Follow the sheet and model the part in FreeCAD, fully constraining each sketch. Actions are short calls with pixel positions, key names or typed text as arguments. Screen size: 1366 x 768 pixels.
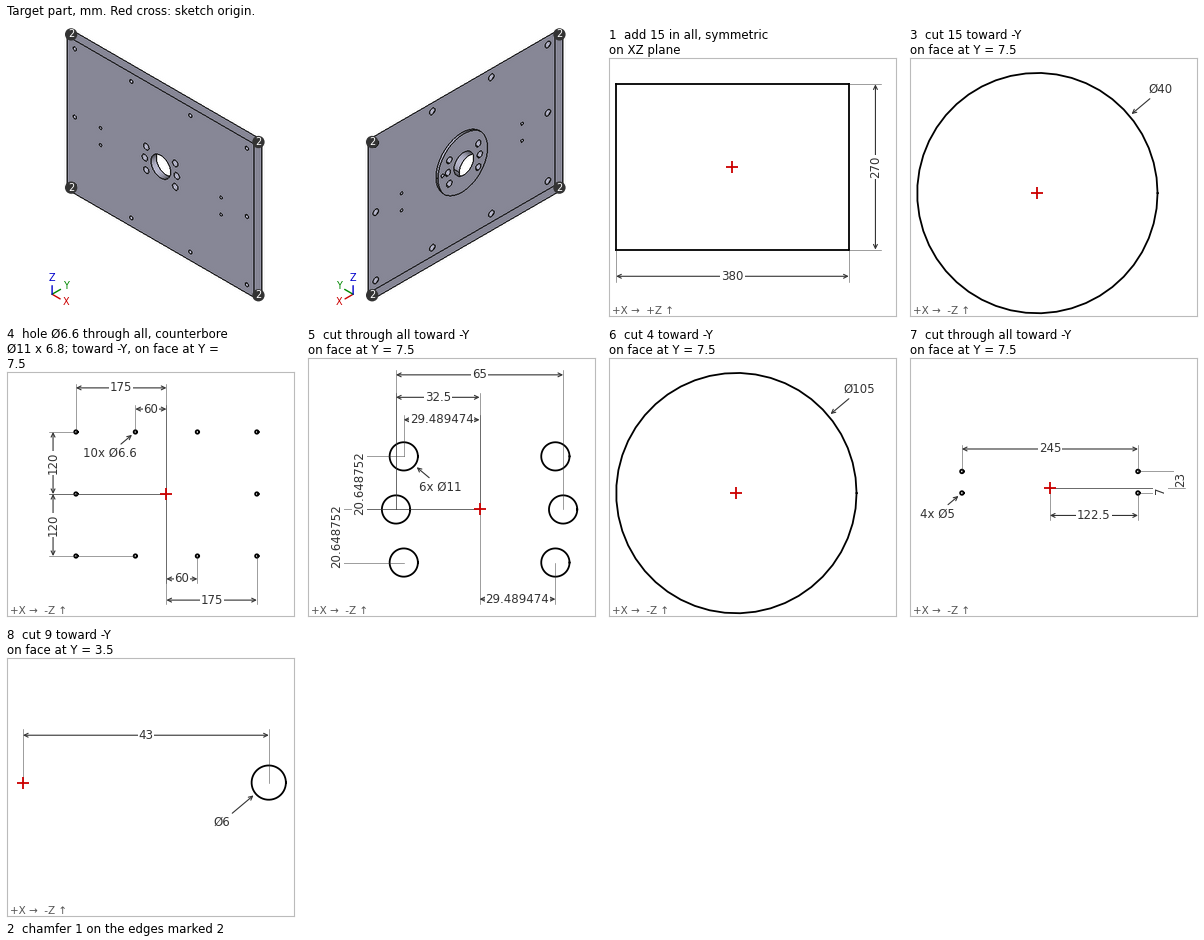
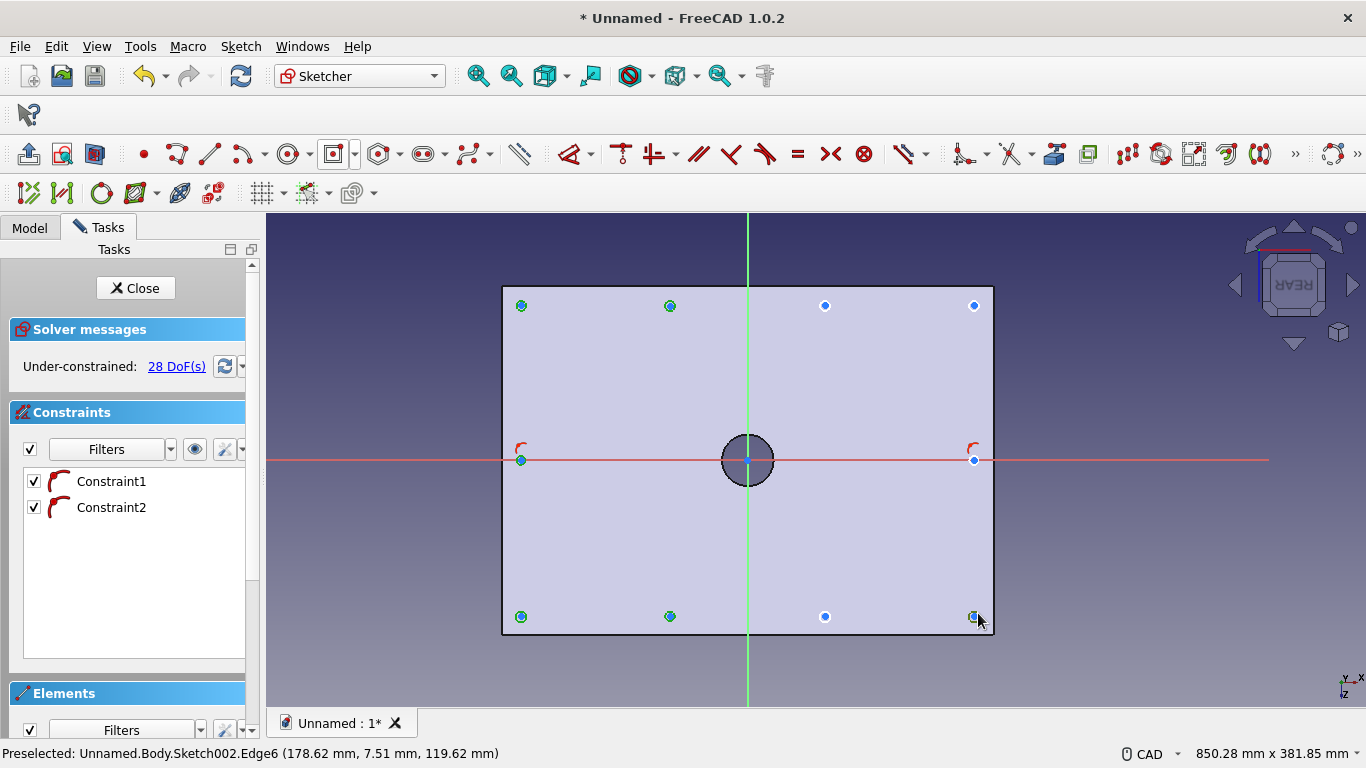
scroll(974, 456, up, 6)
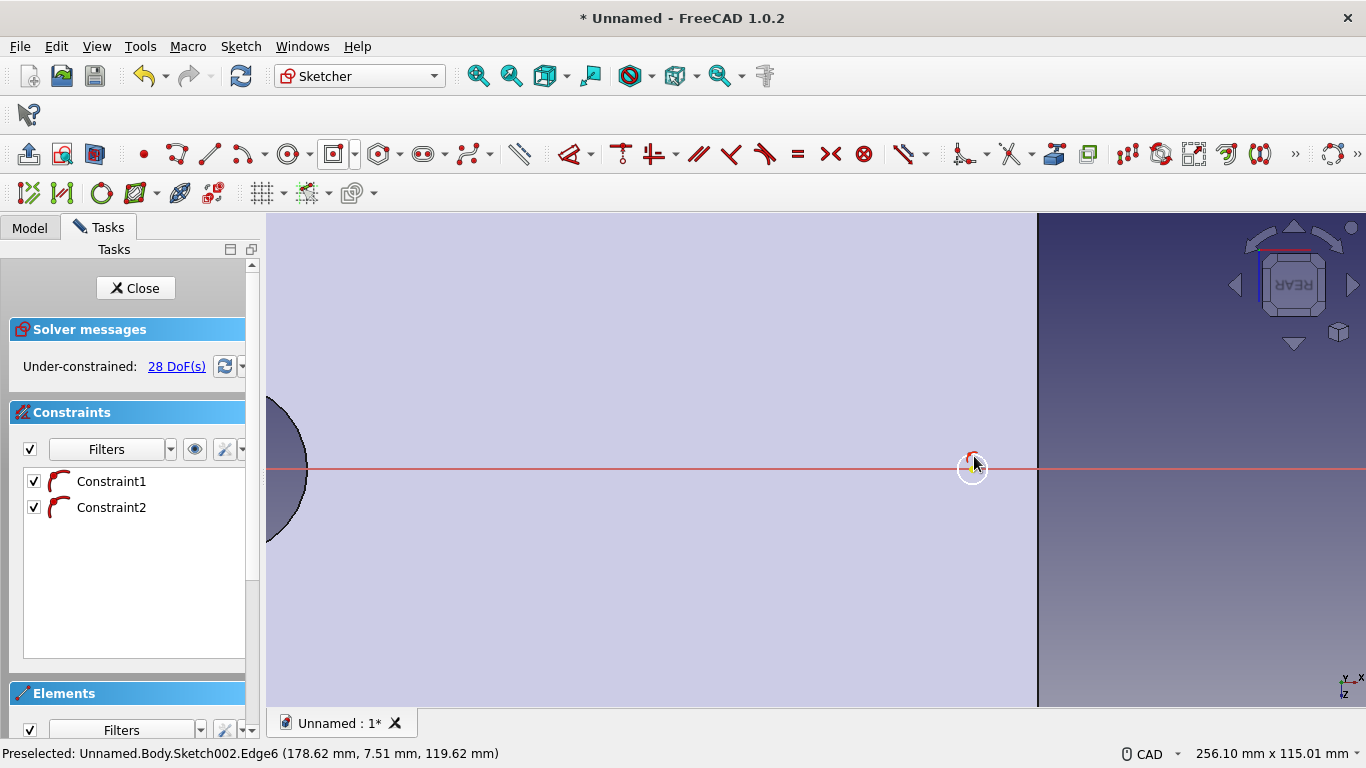
click(958, 469)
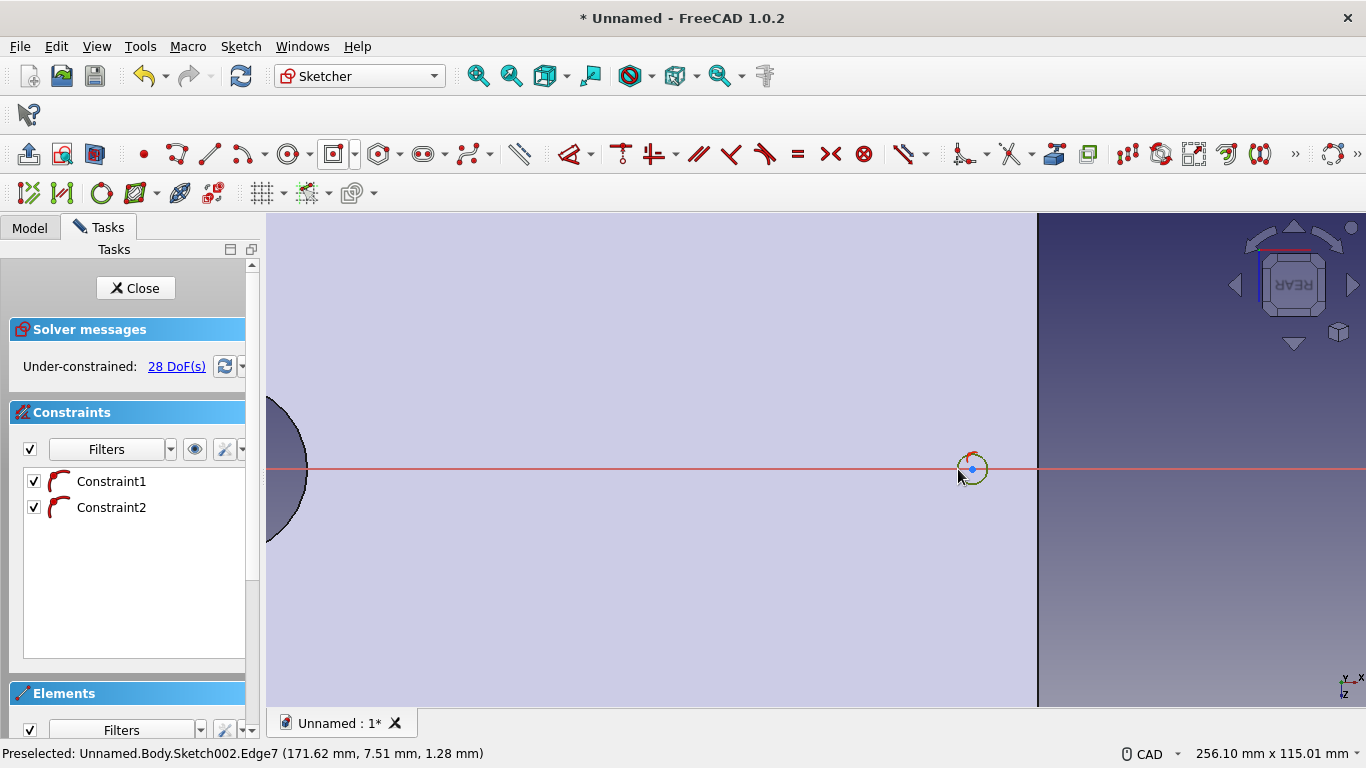
scroll(974, 456, down, 6)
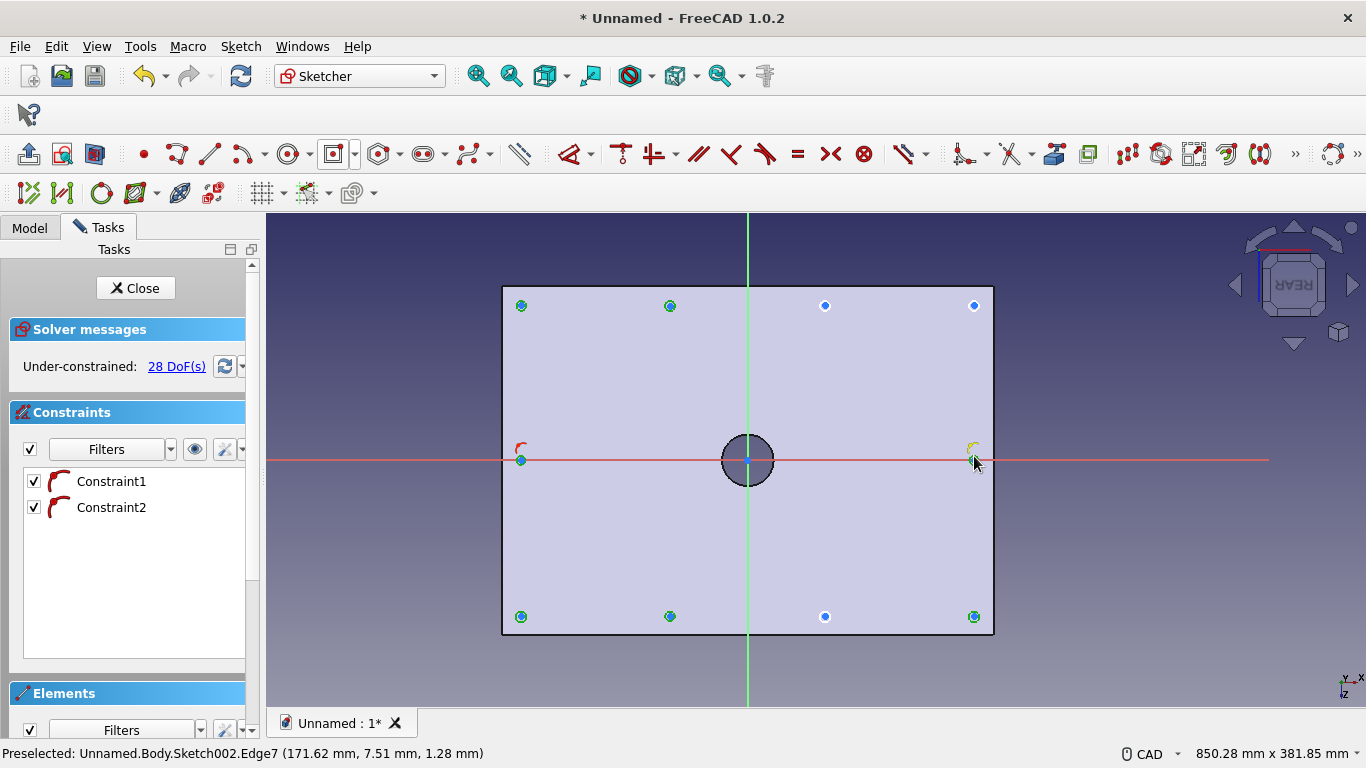
scroll(829, 613, up, 5)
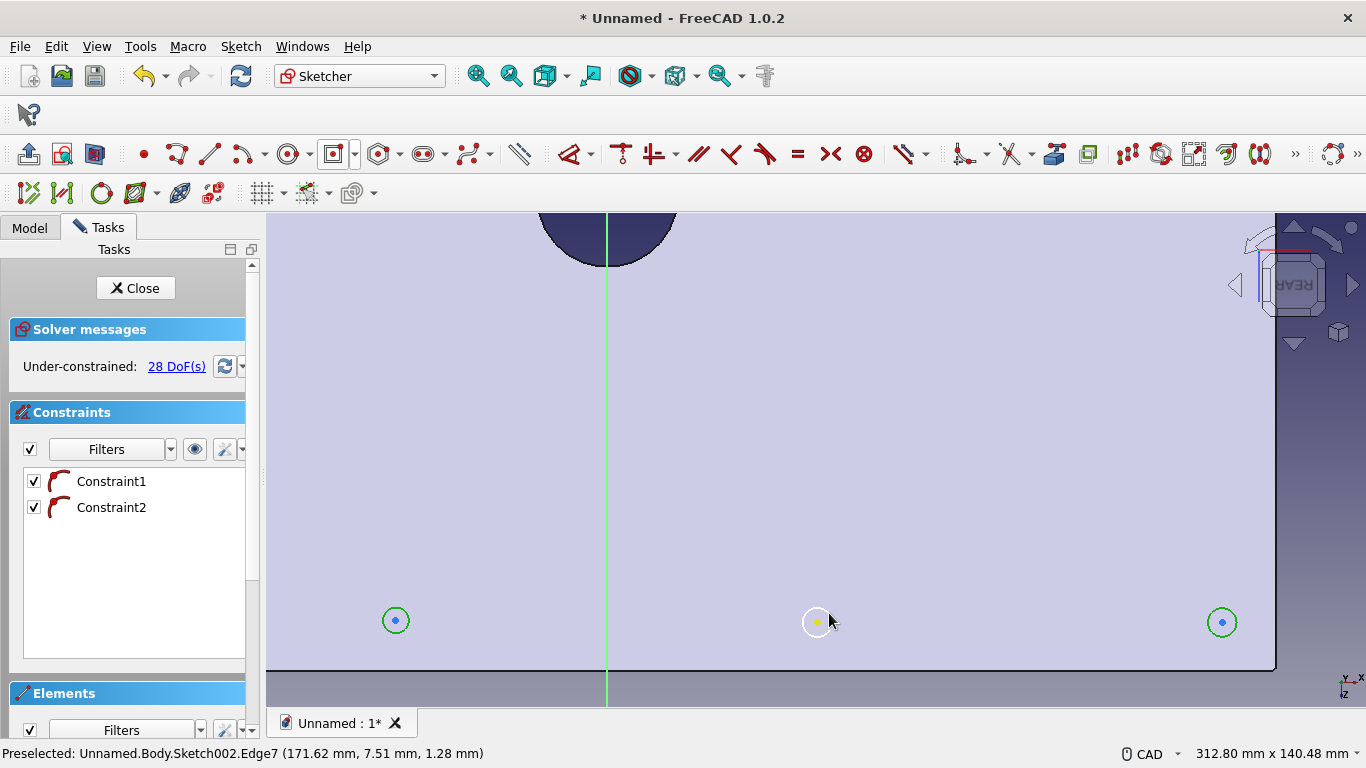
click(827, 612)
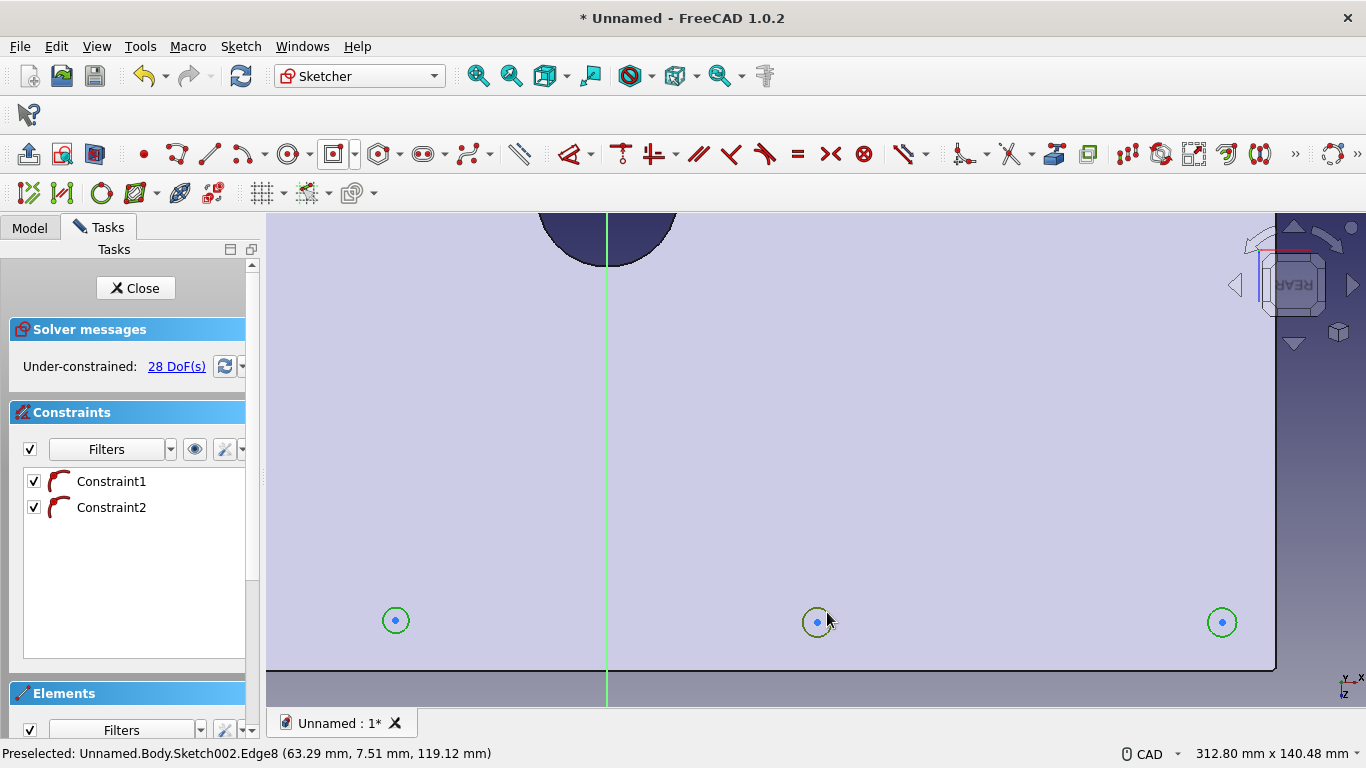
scroll(829, 613, down, 5)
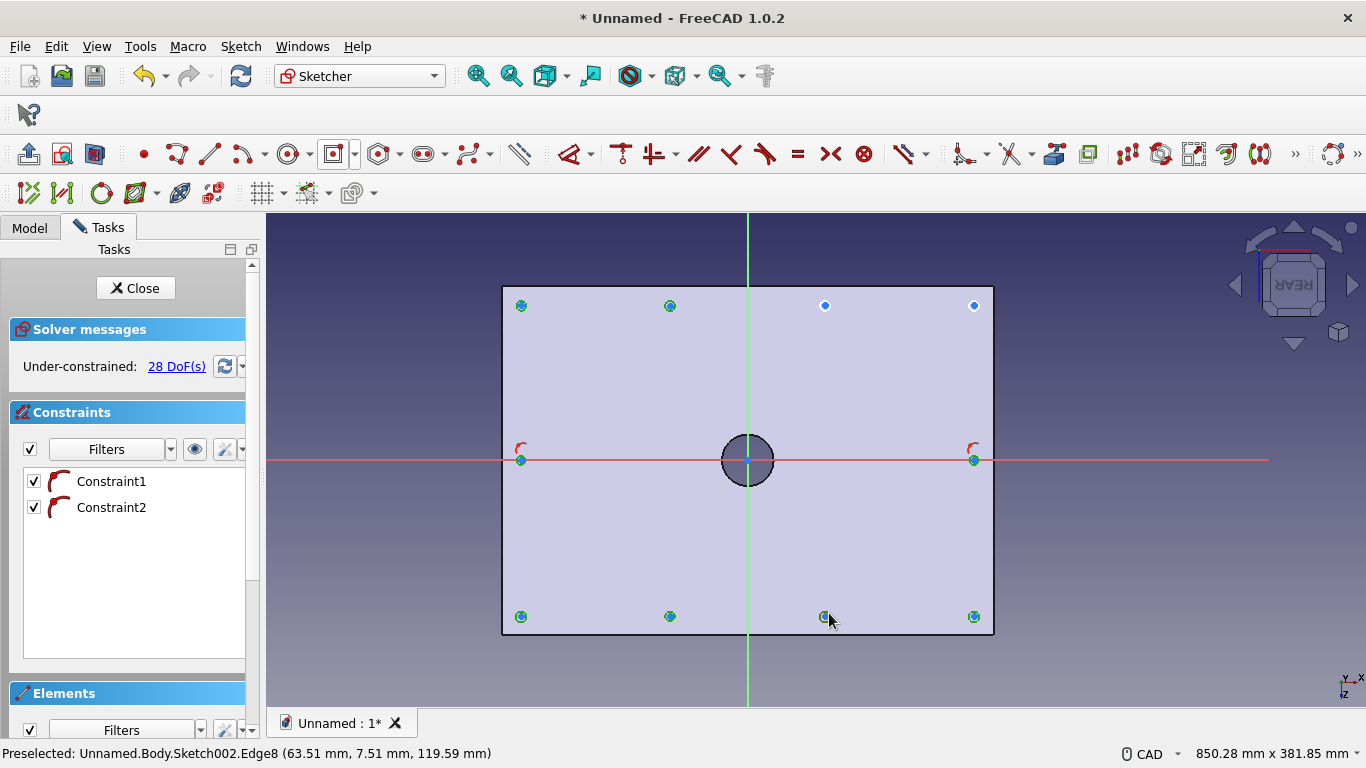
scroll(828, 302, up, 6)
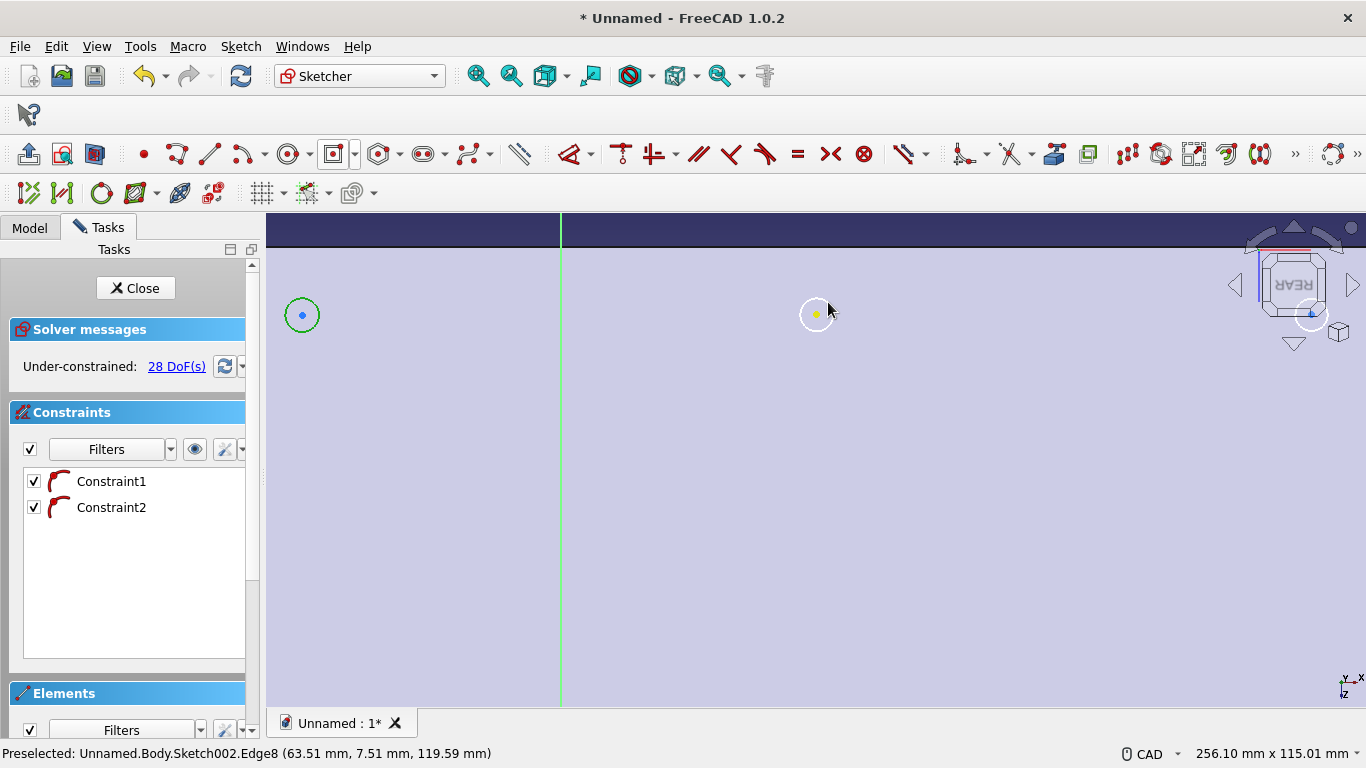
click(828, 303)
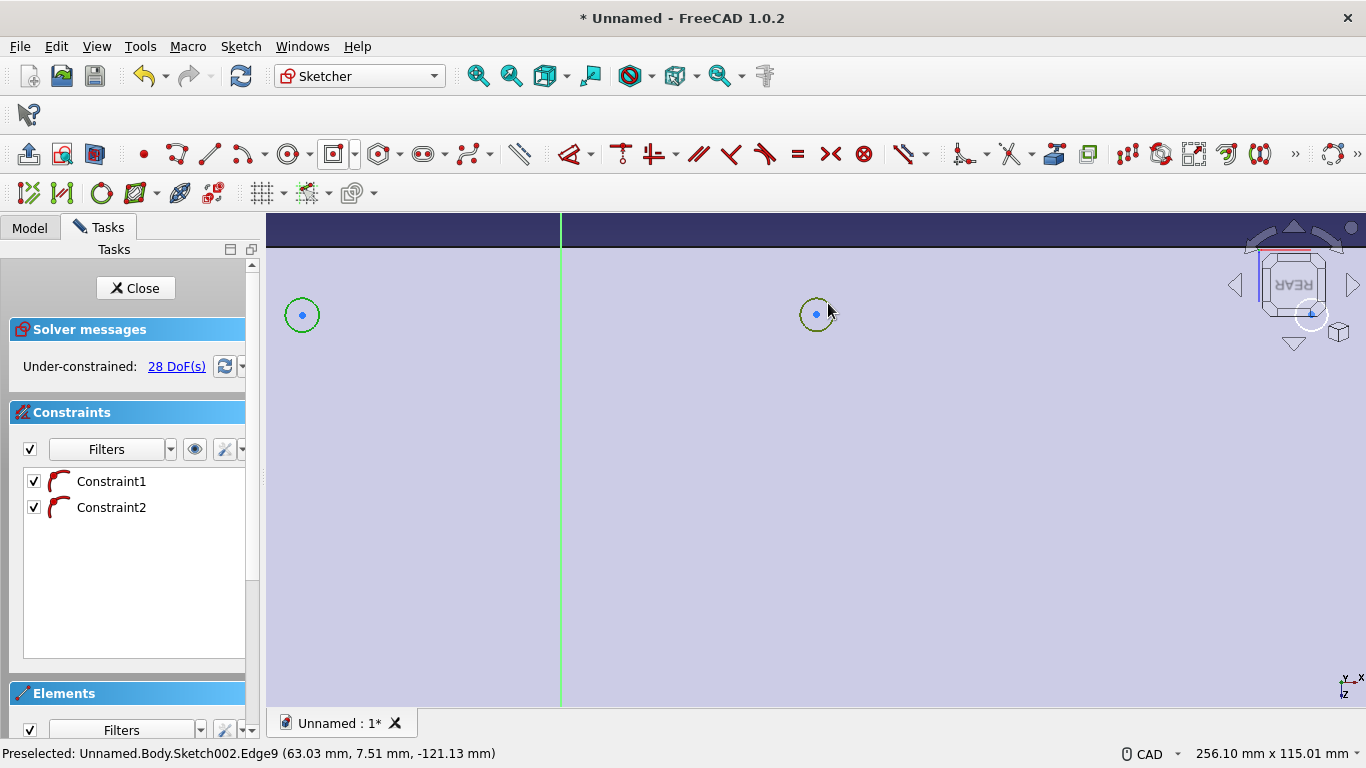
scroll(828, 302, down, 6)